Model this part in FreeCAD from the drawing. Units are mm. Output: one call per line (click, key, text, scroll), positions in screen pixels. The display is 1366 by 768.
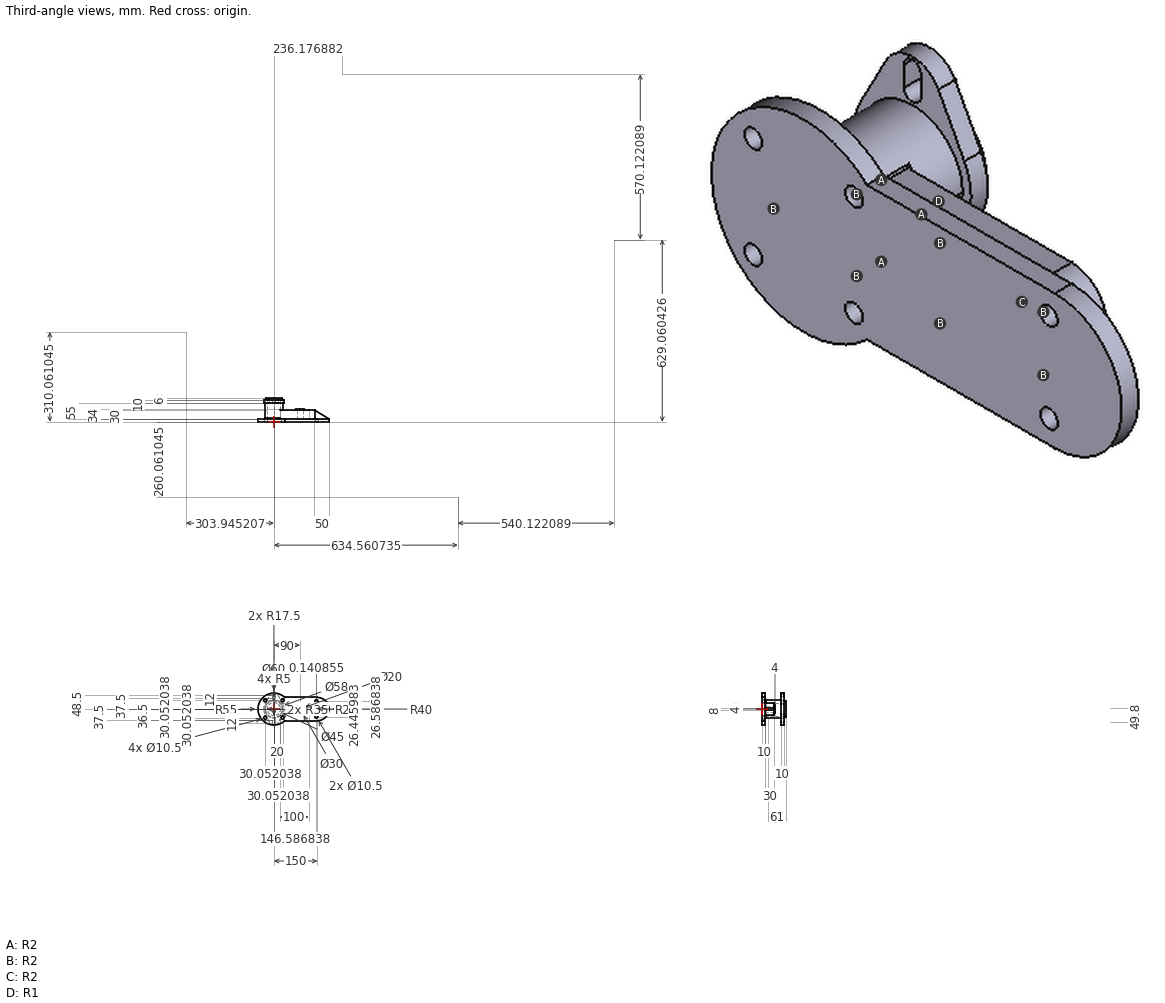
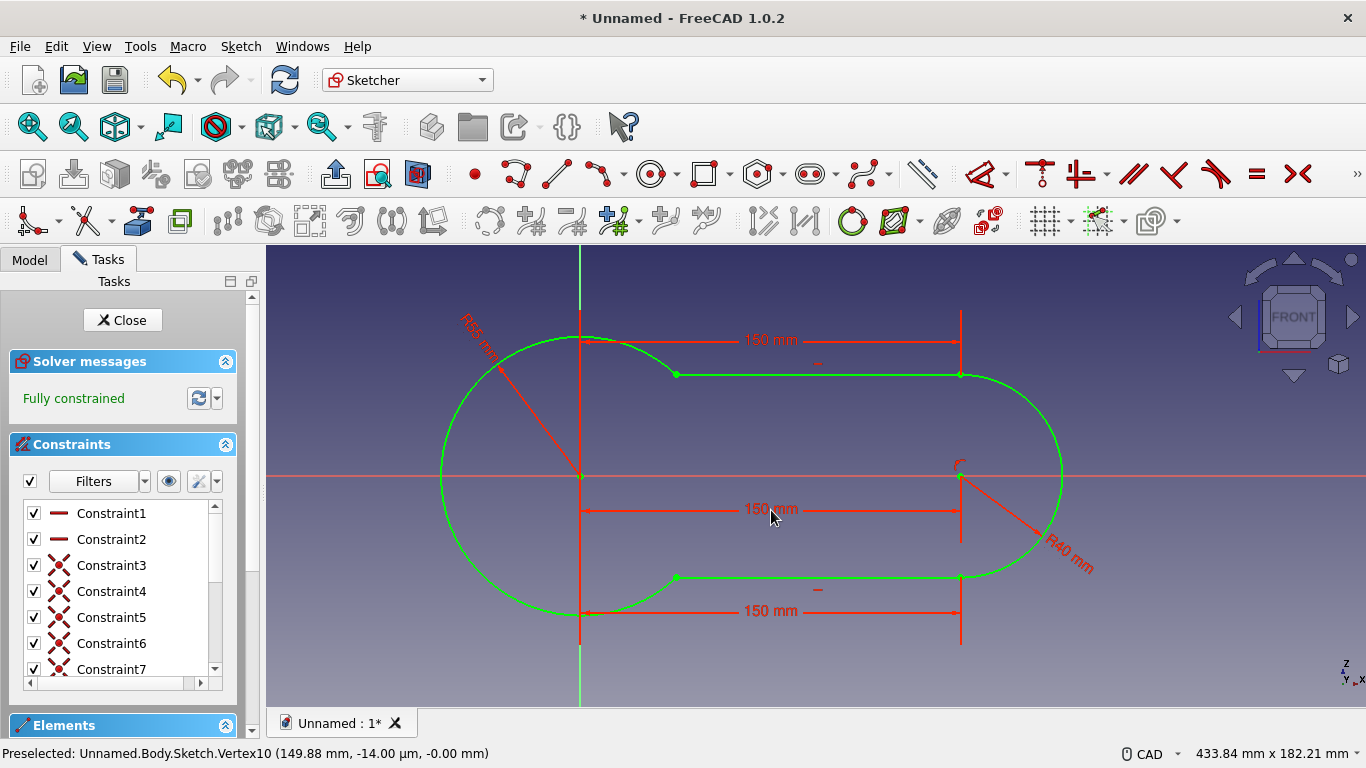
click(123, 320)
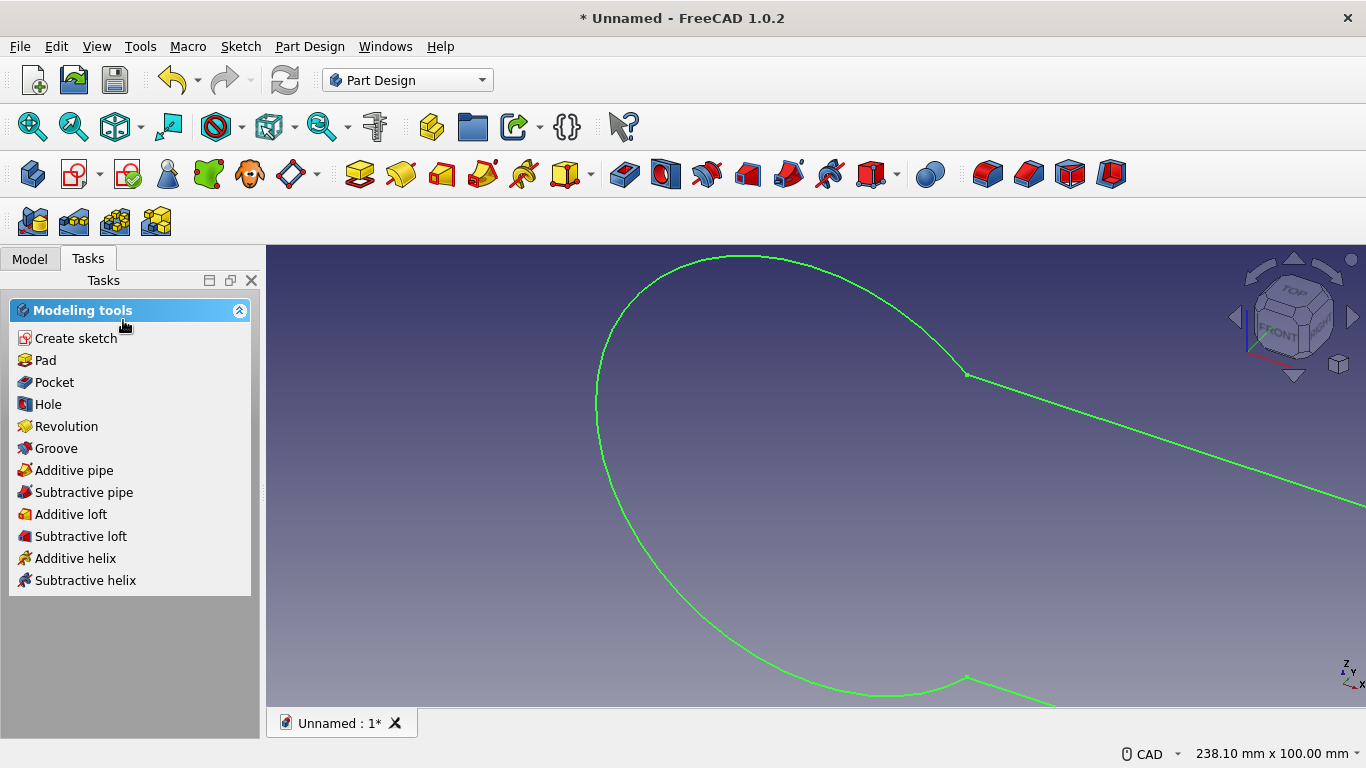
click(360, 174)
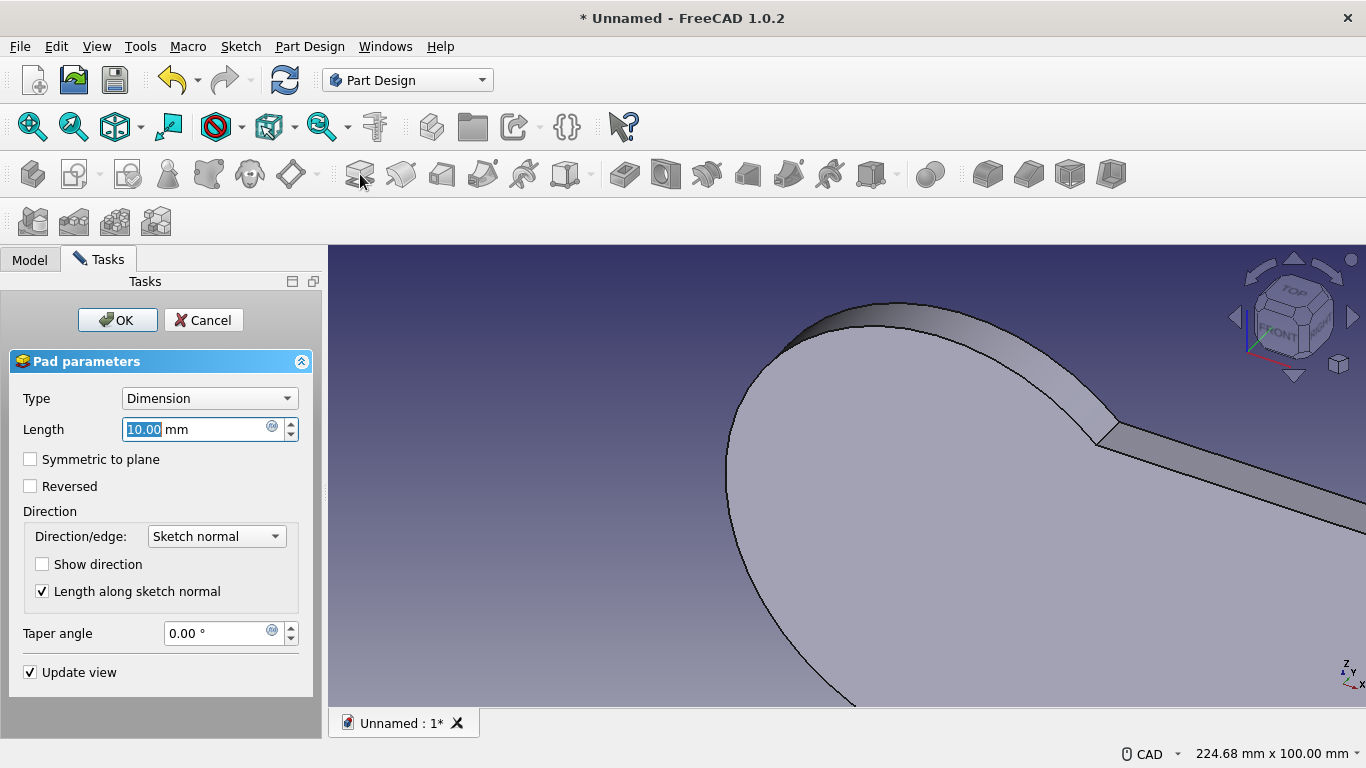
text(10)
key(Tab)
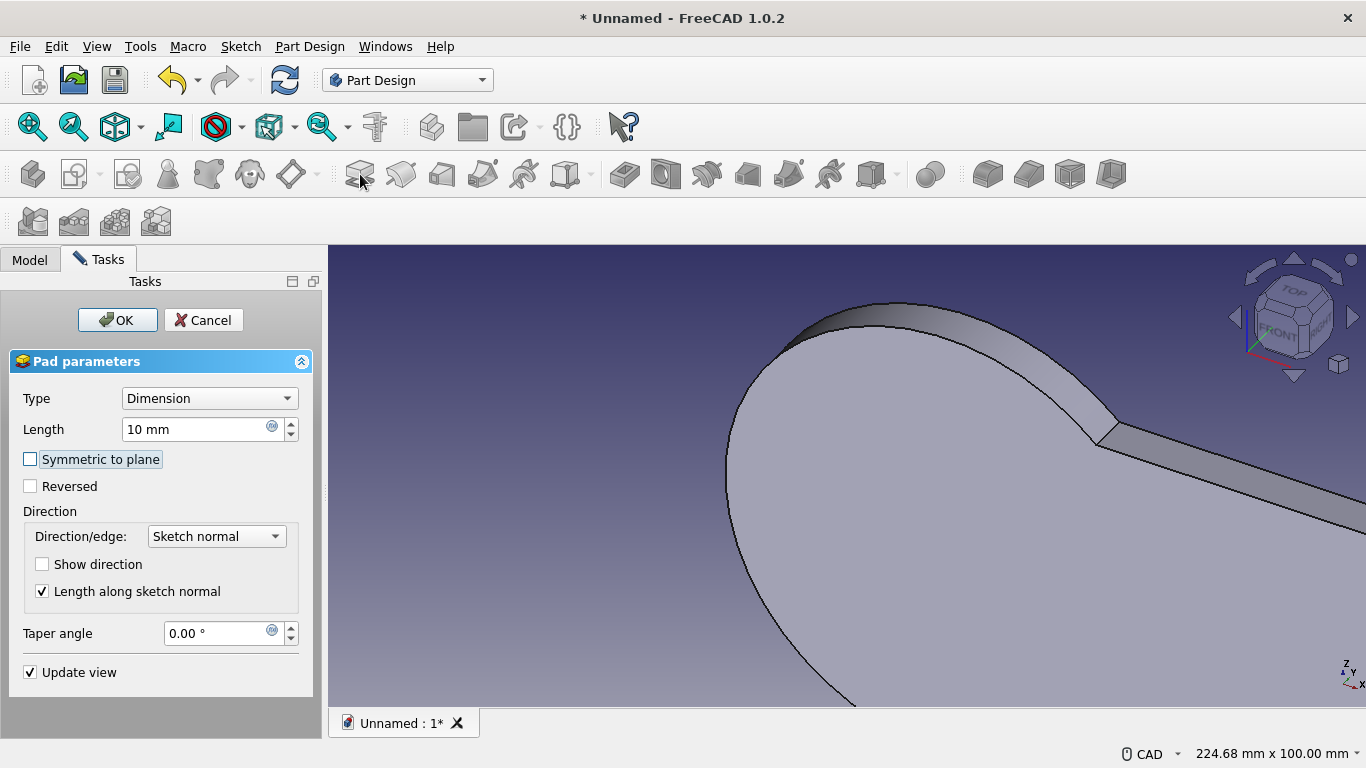
click(31, 486)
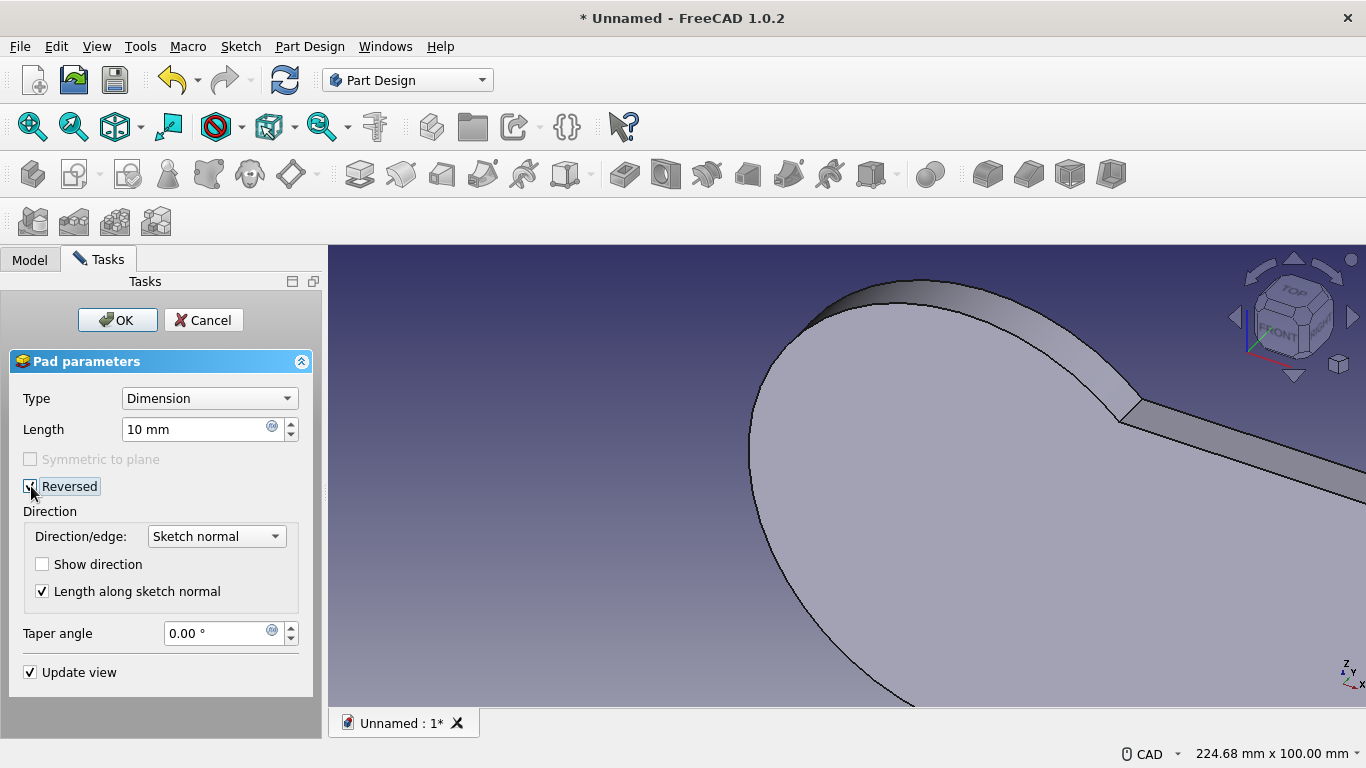
click(118, 320)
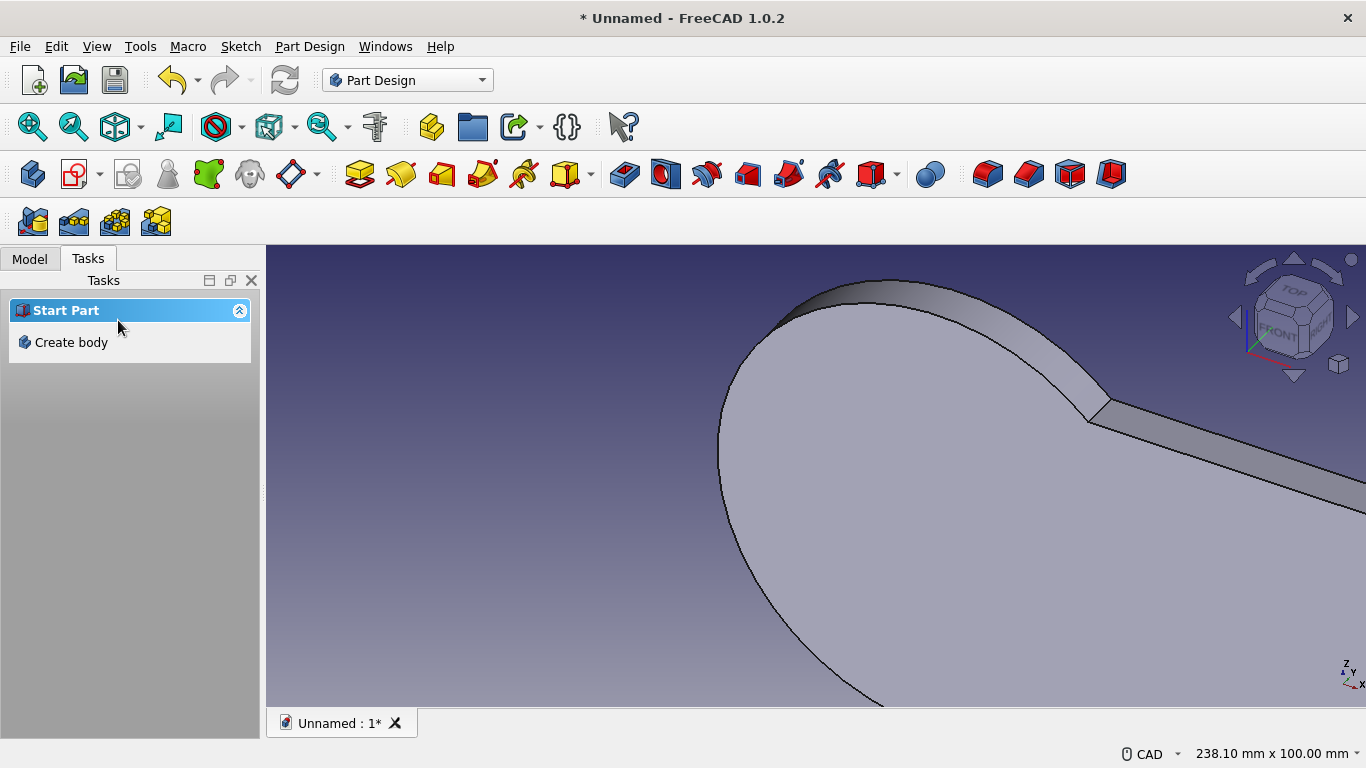
key(v)
key(f)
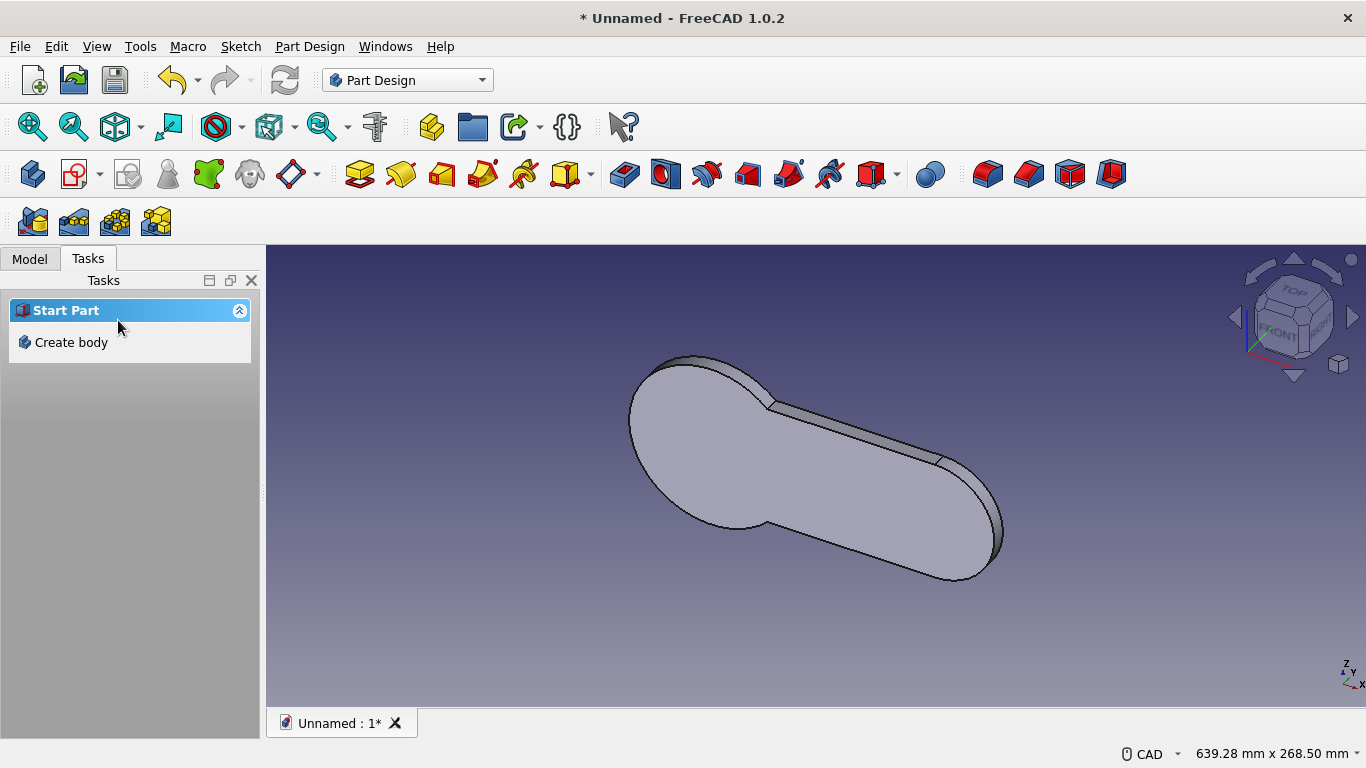
key(4)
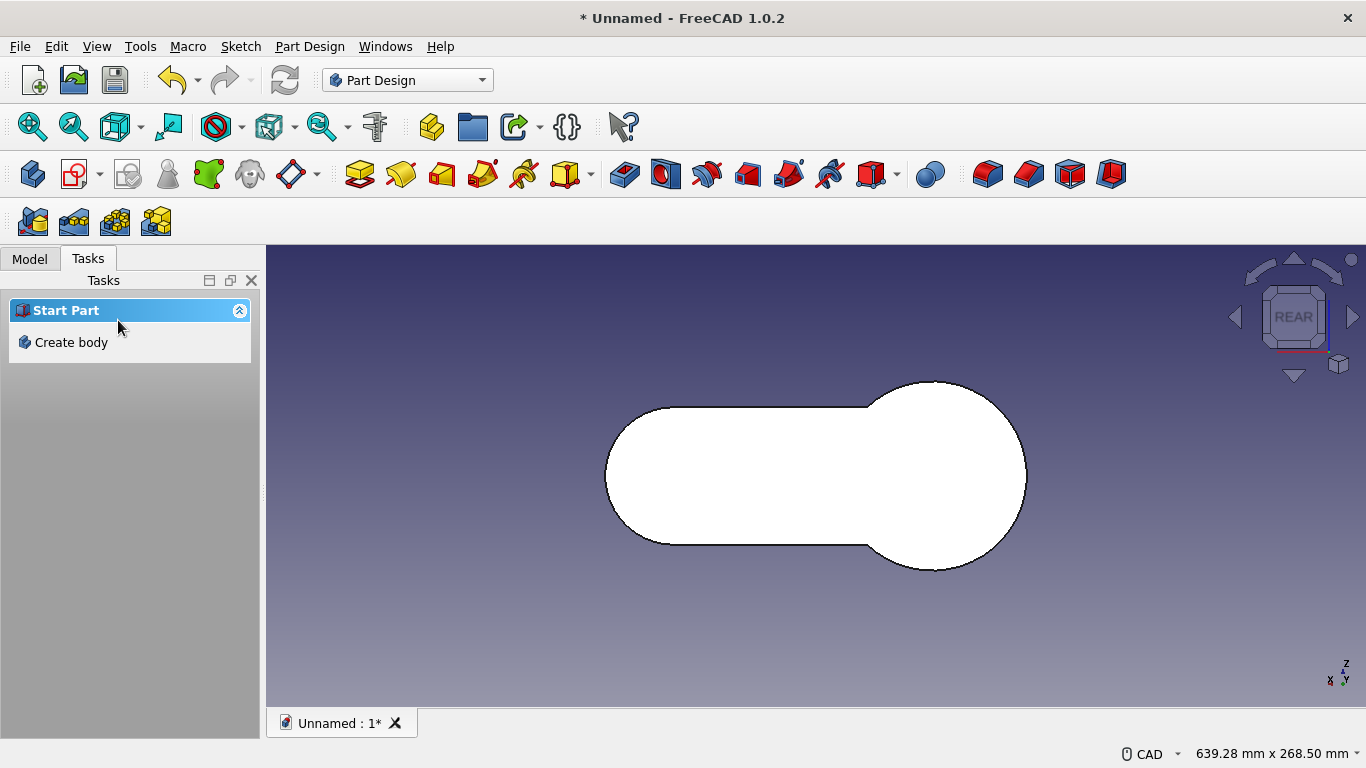
key(v)
key(f)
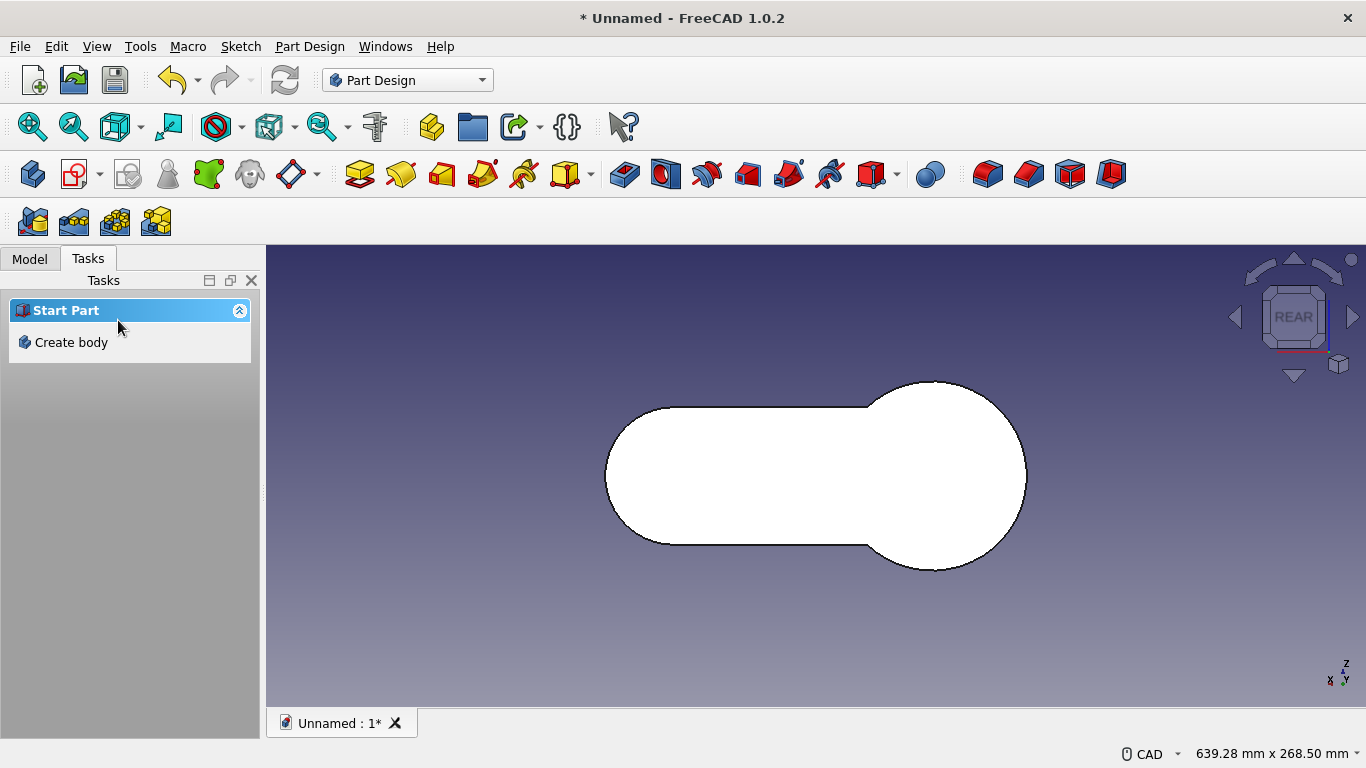
click(936, 475)